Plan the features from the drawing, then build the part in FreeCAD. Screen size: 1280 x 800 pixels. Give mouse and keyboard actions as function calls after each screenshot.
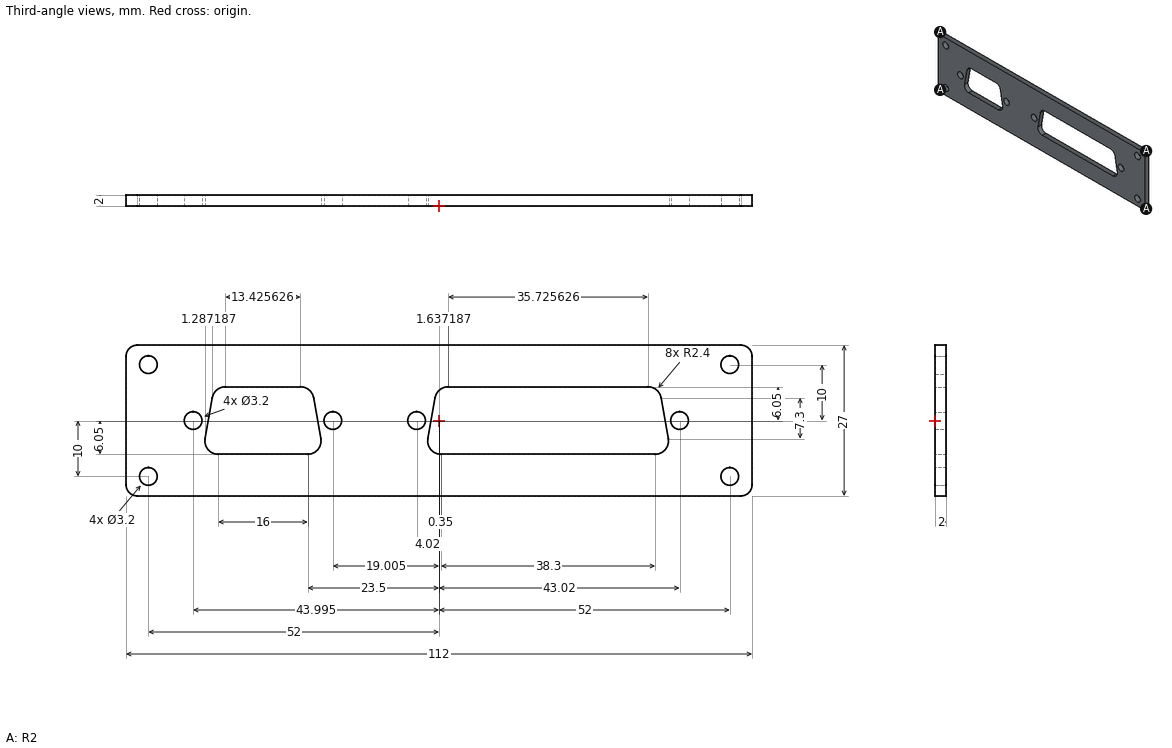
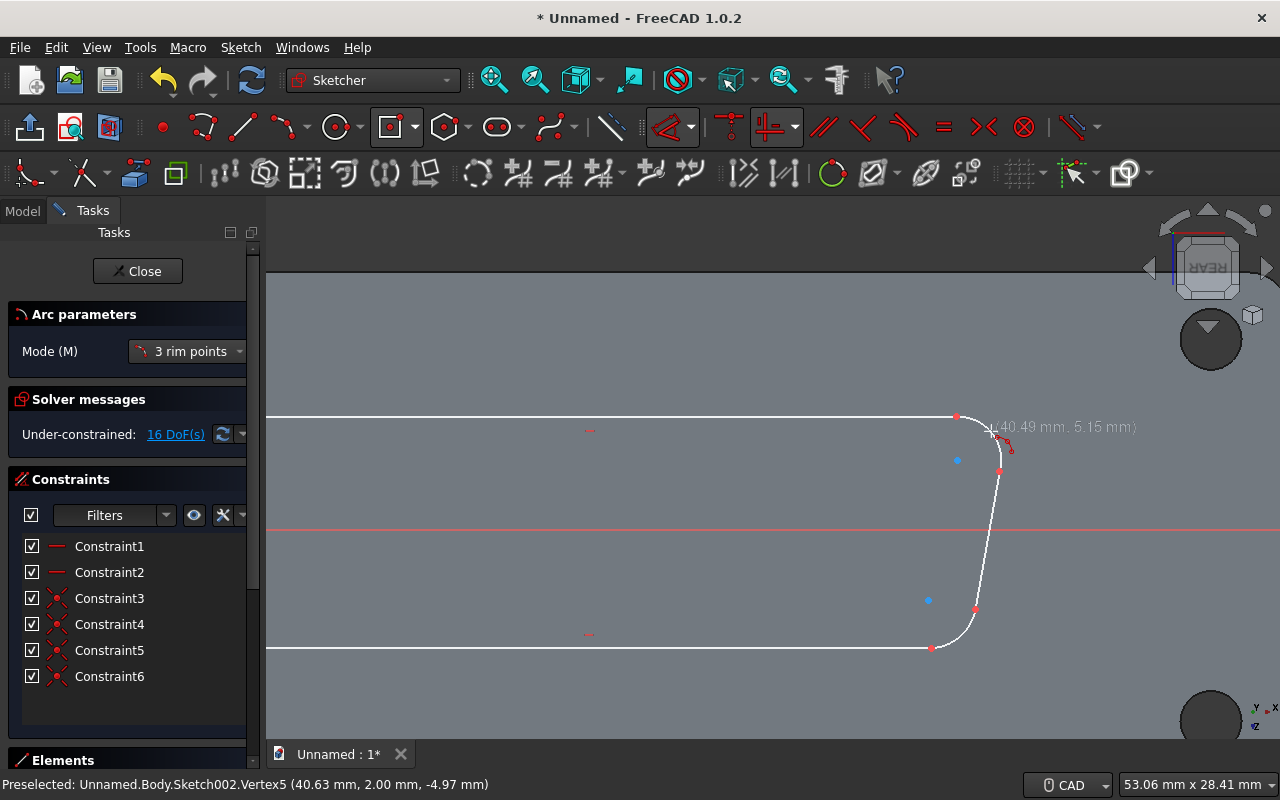
scroll(993, 431, down, 5)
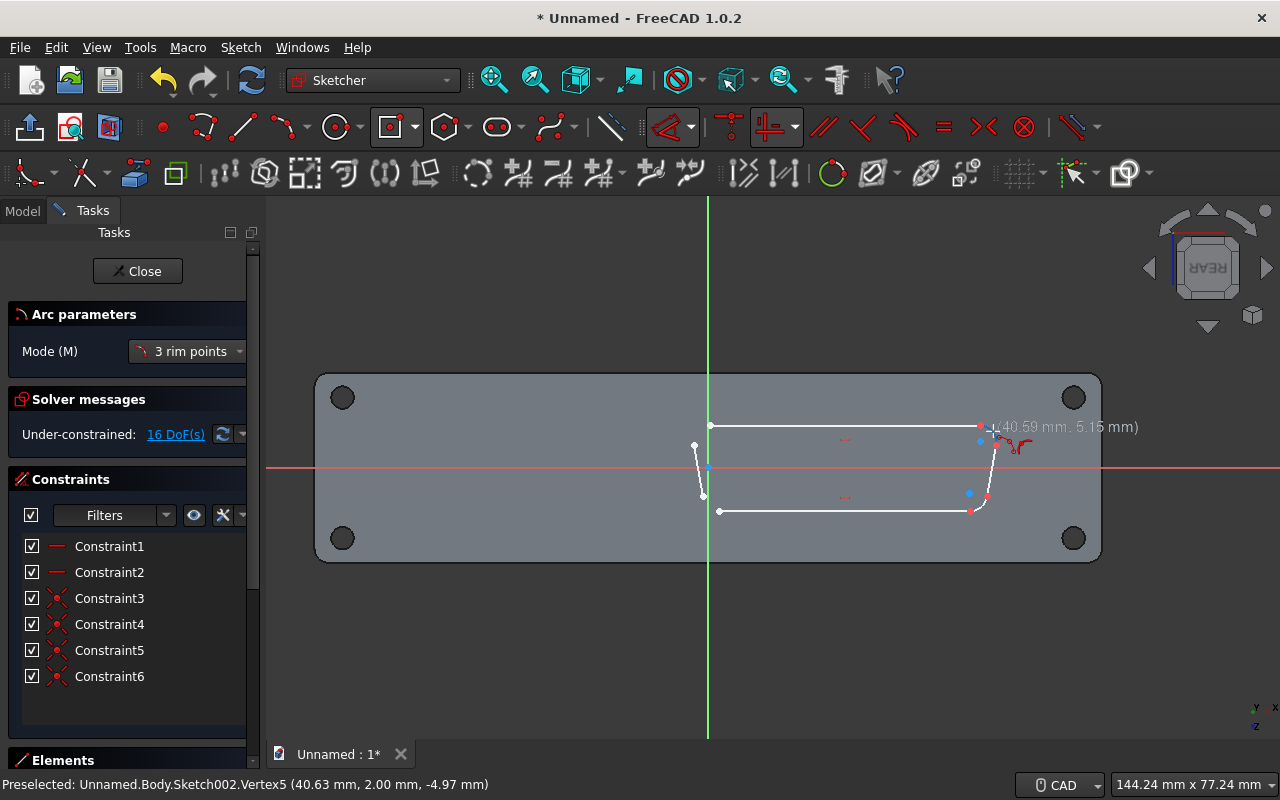
scroll(711, 425, up, 10)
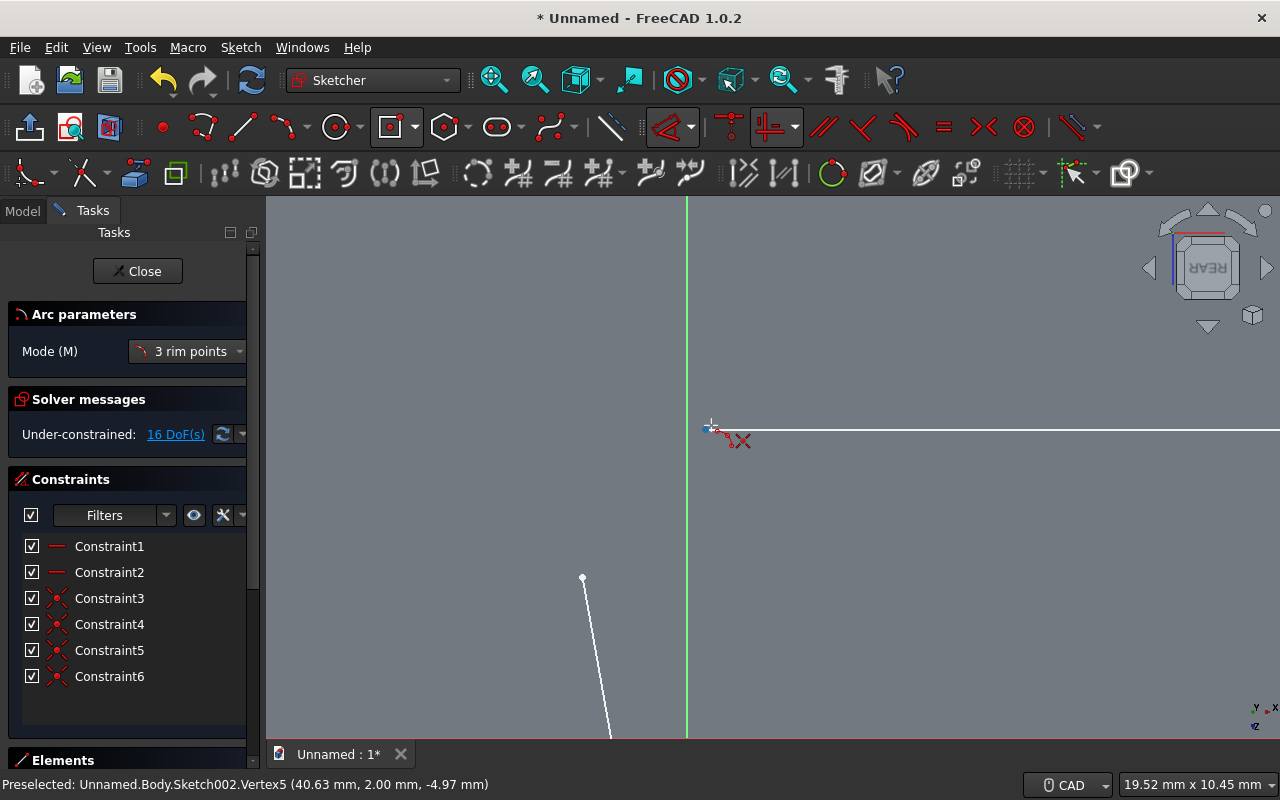
click(705, 430)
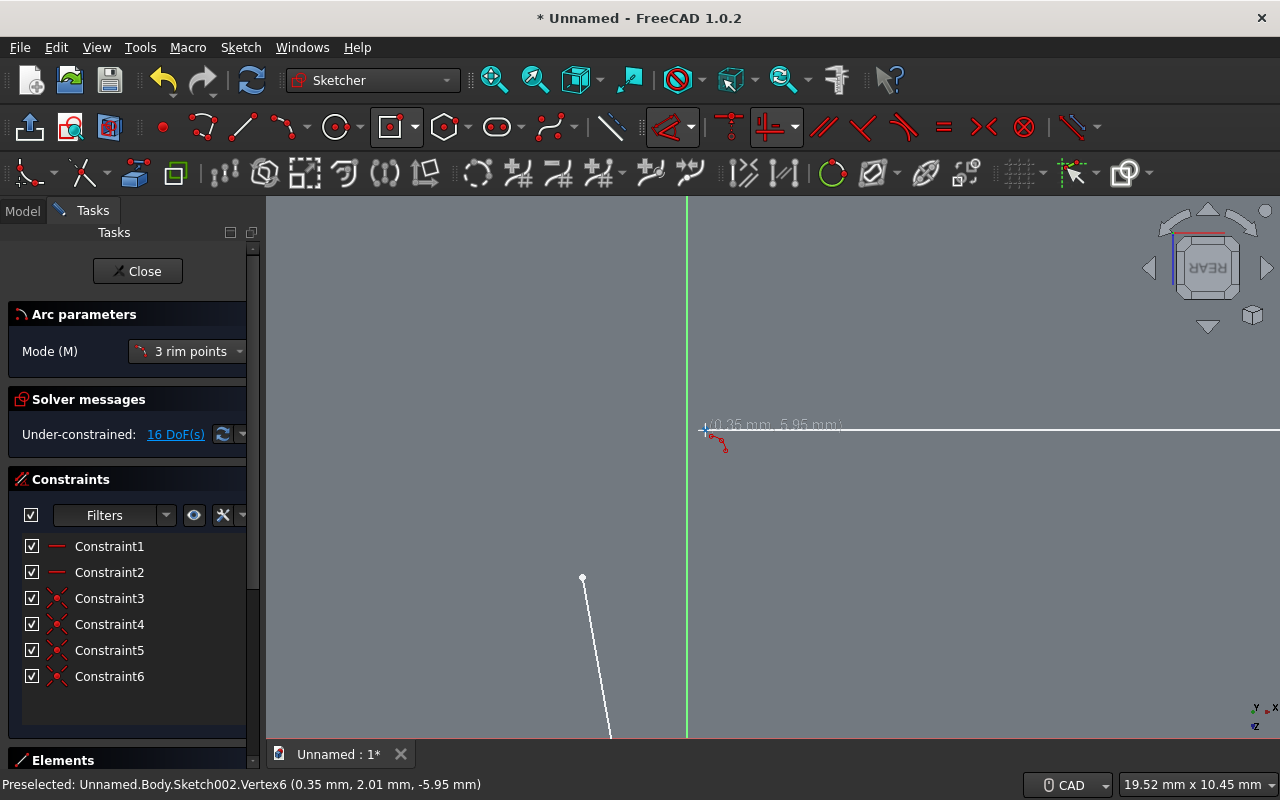
scroll(711, 425, down, 10)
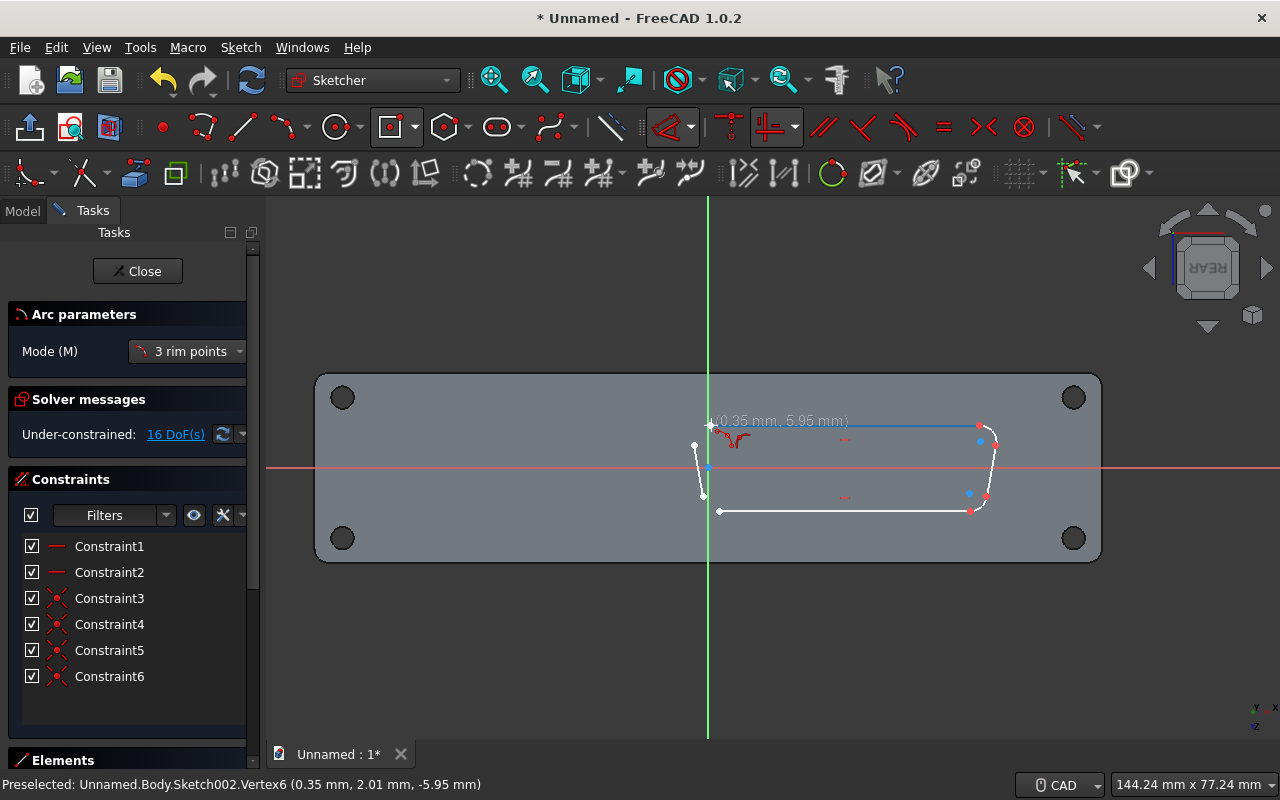
click(694, 446)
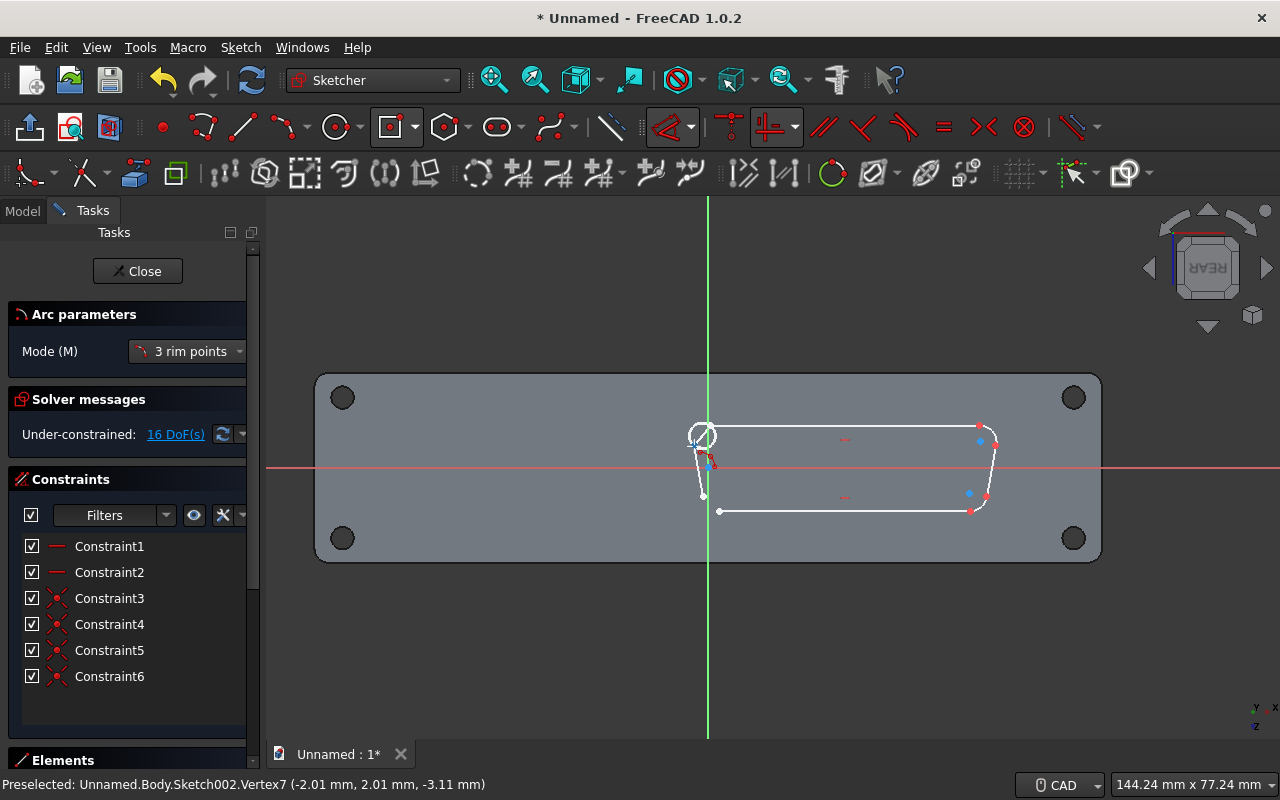
scroll(698, 431, up, 5)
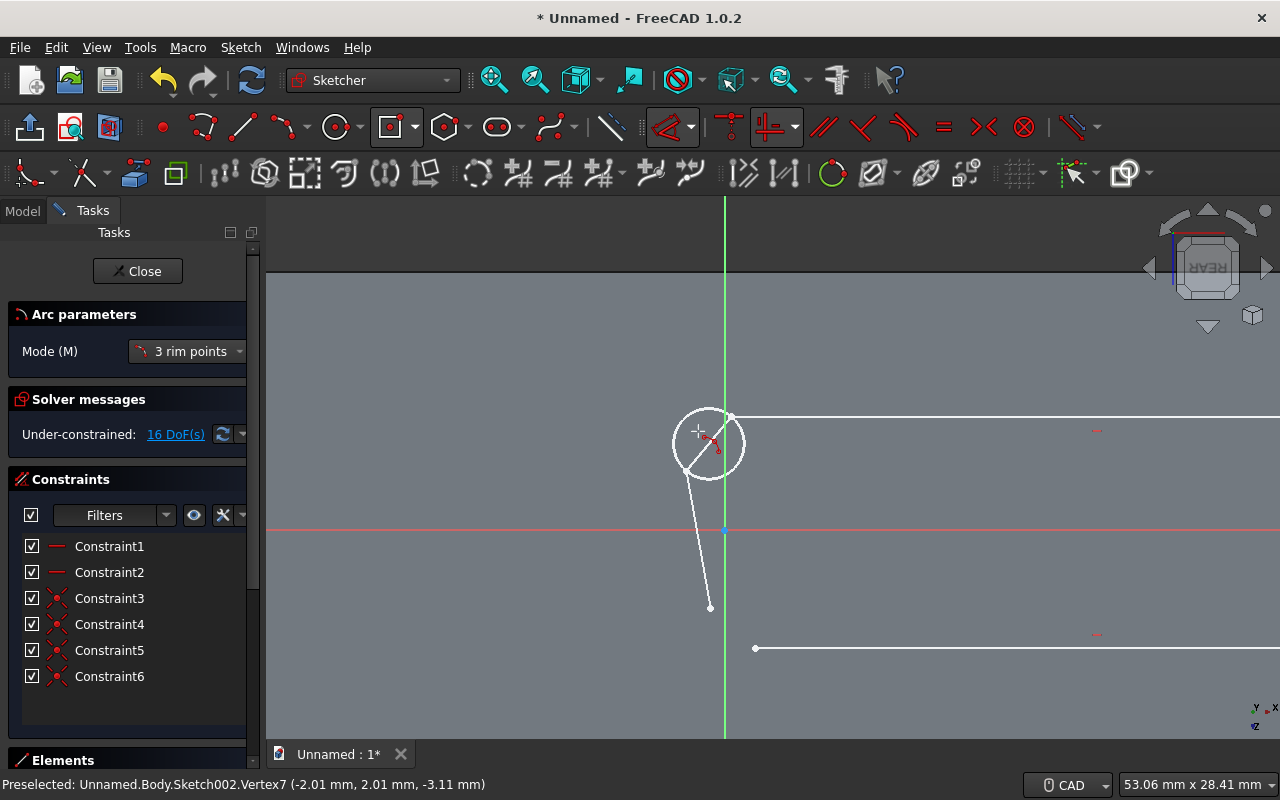
click(696, 431)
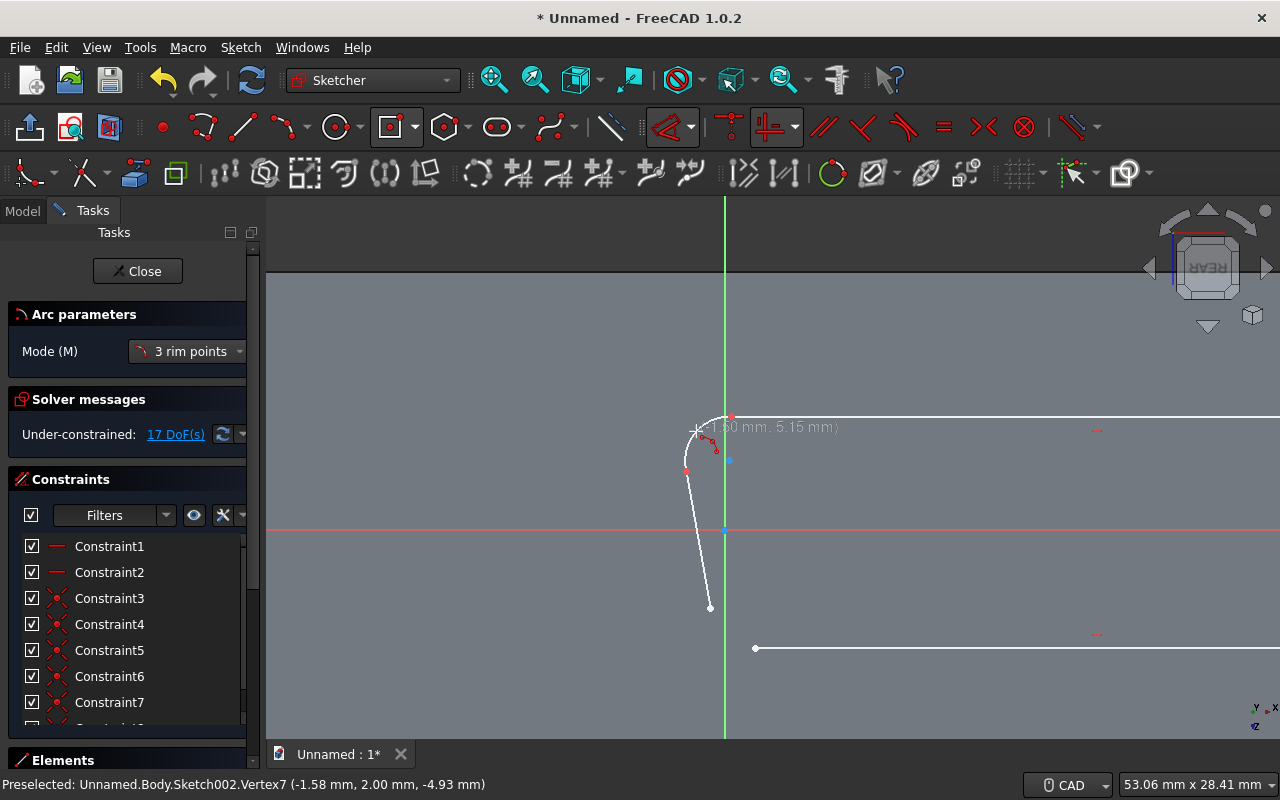
click(711, 609)
click(756, 648)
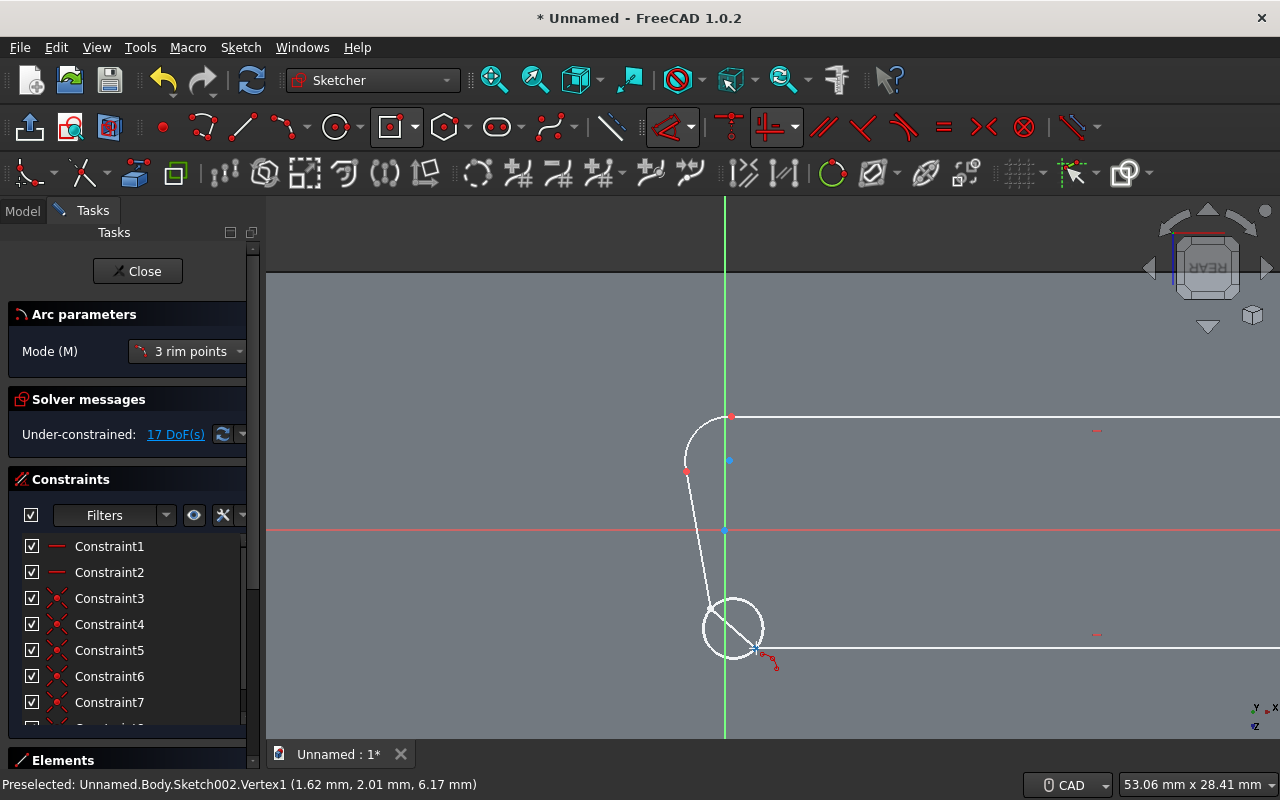
scroll(737, 642, up, 3)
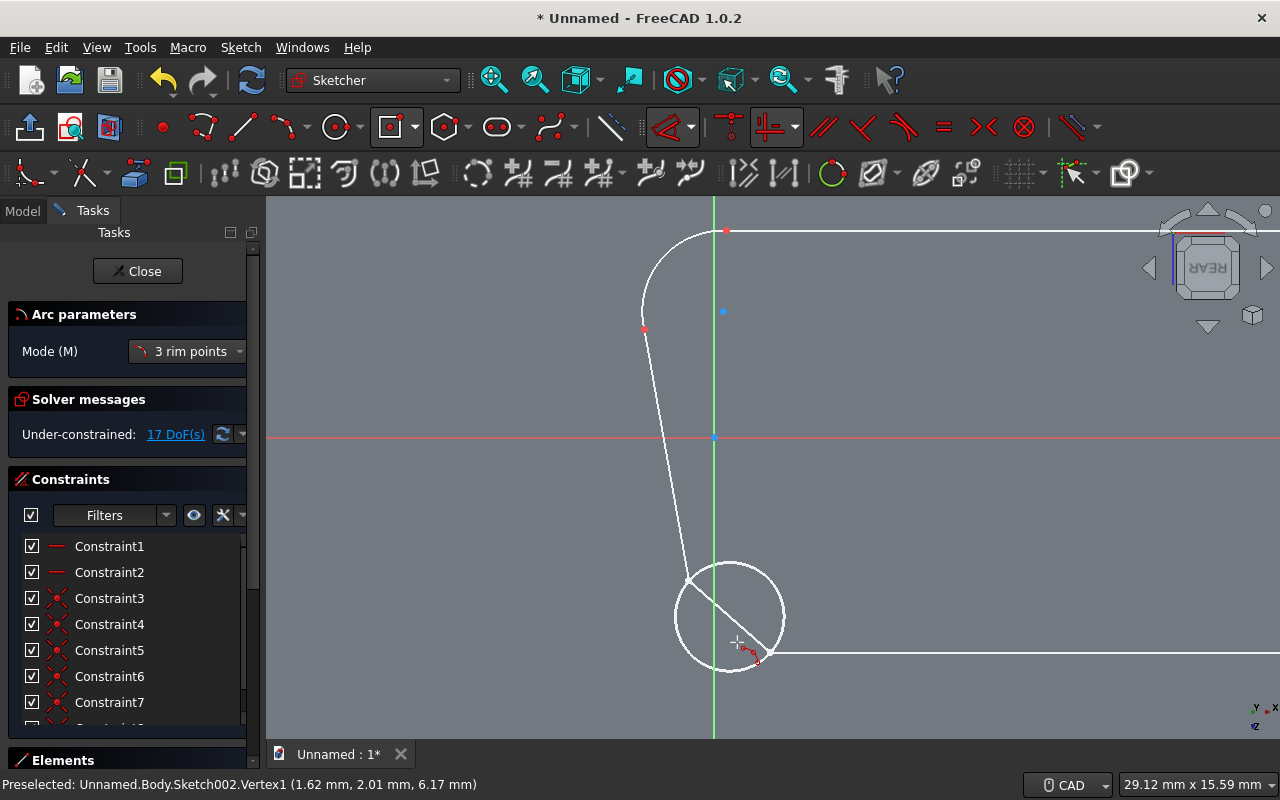
click(737, 641)